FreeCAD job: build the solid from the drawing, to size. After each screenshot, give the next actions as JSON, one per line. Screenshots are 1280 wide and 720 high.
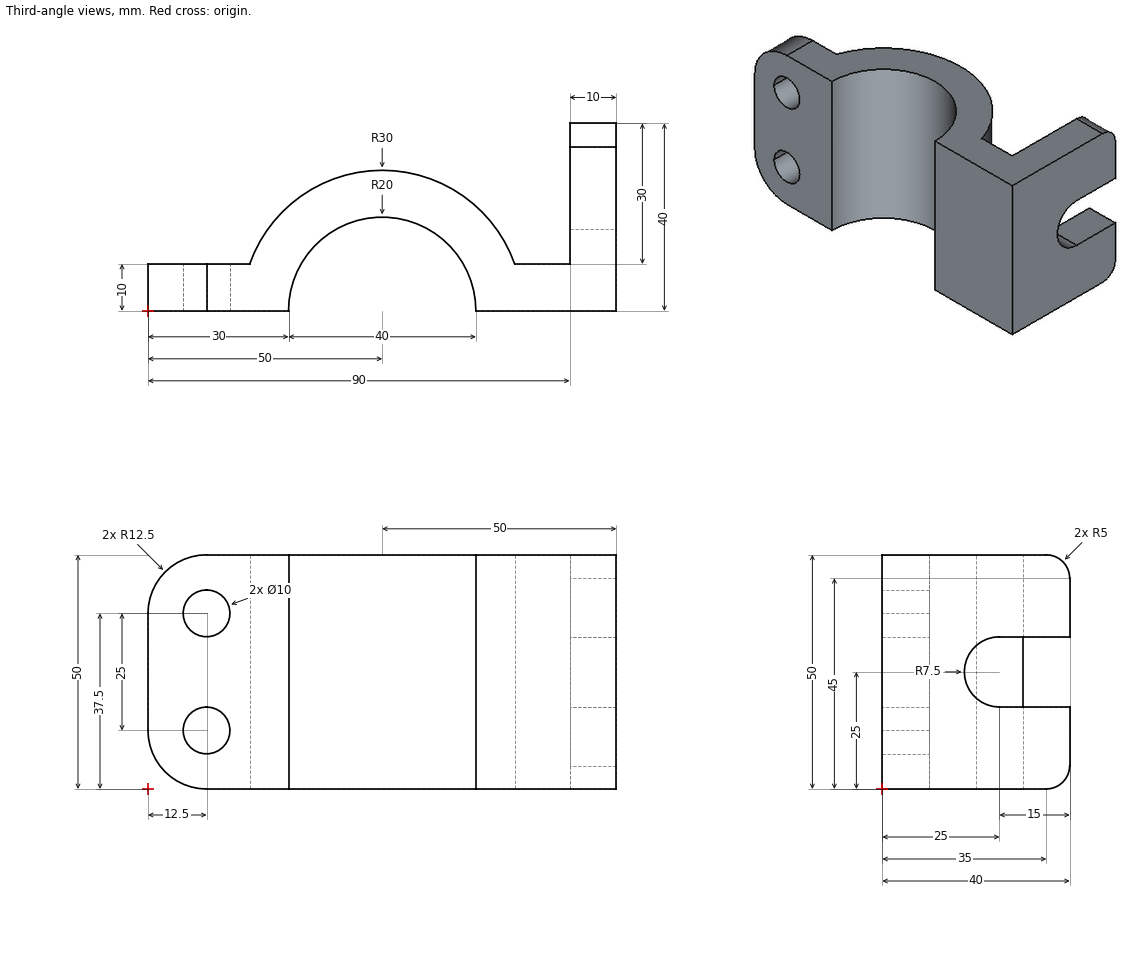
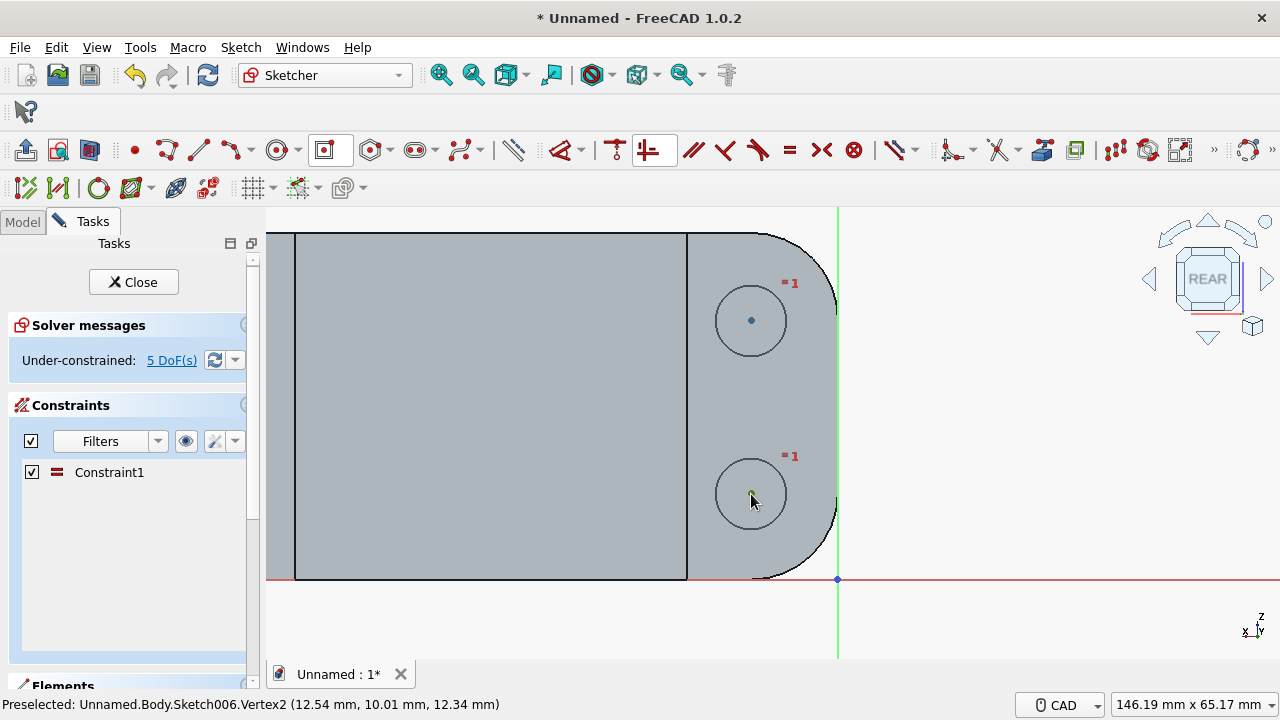
{"action": "key", "text": "v"}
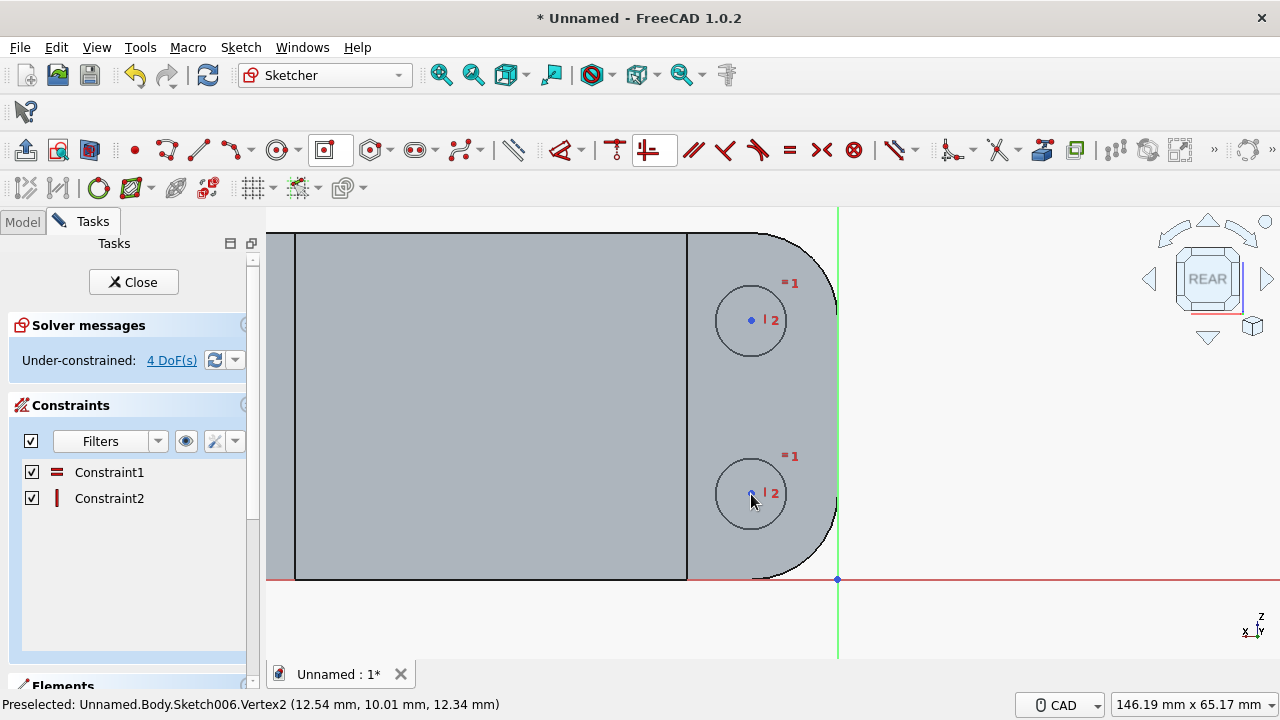
{"action": "left_click", "coordinate": [560, 150]}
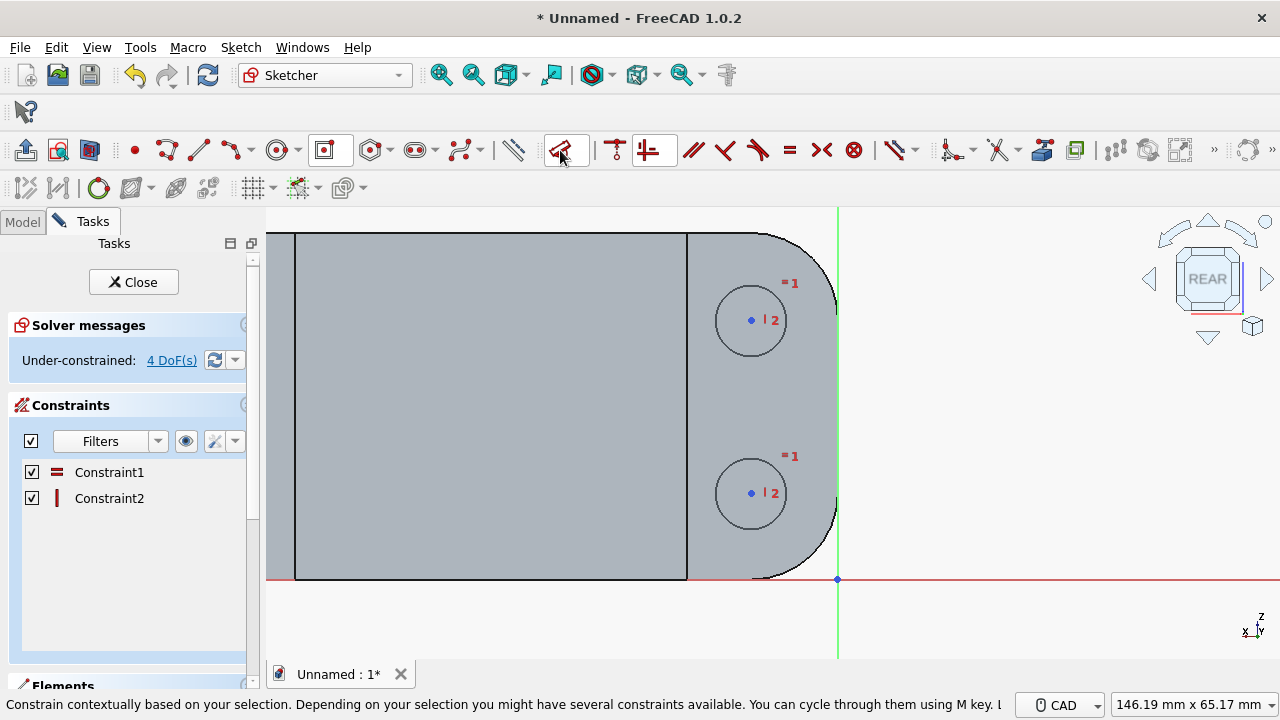
{"action": "left_click", "coordinate": [776, 296]}
{"action": "left_click", "coordinate": [799, 273]}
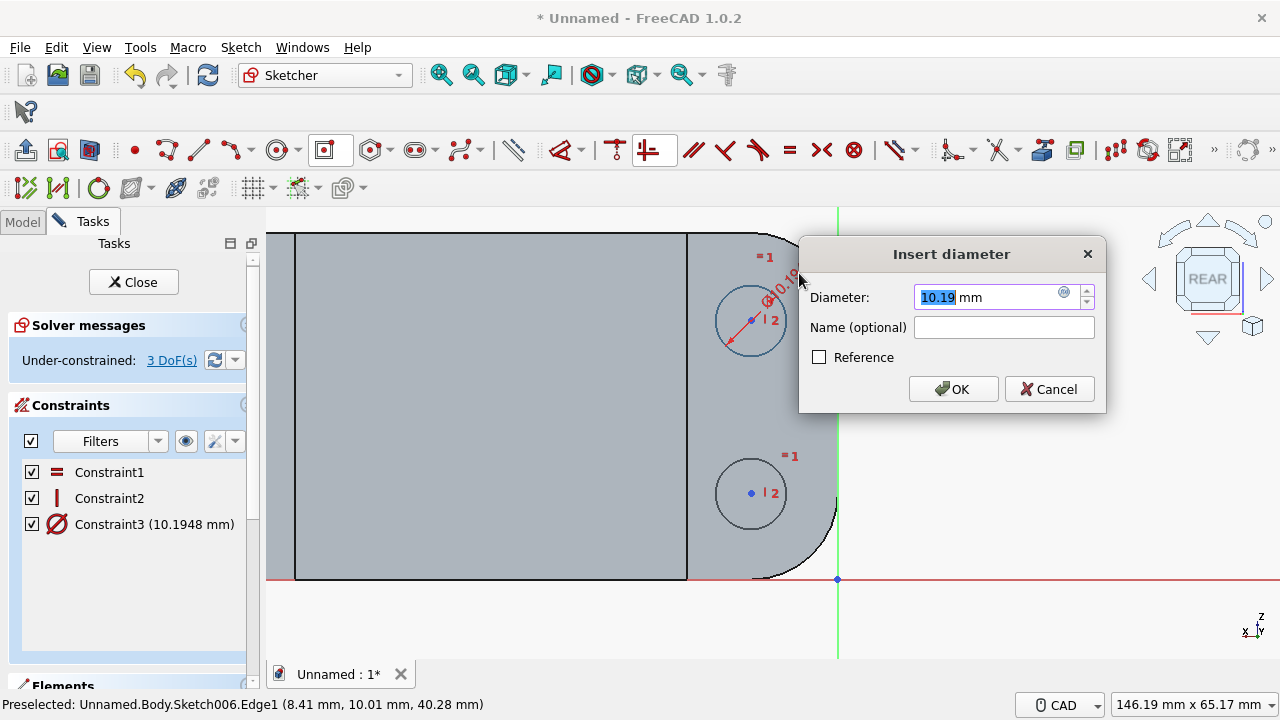
{"action": "type", "text": "10"}
{"action": "key", "text": "Return"}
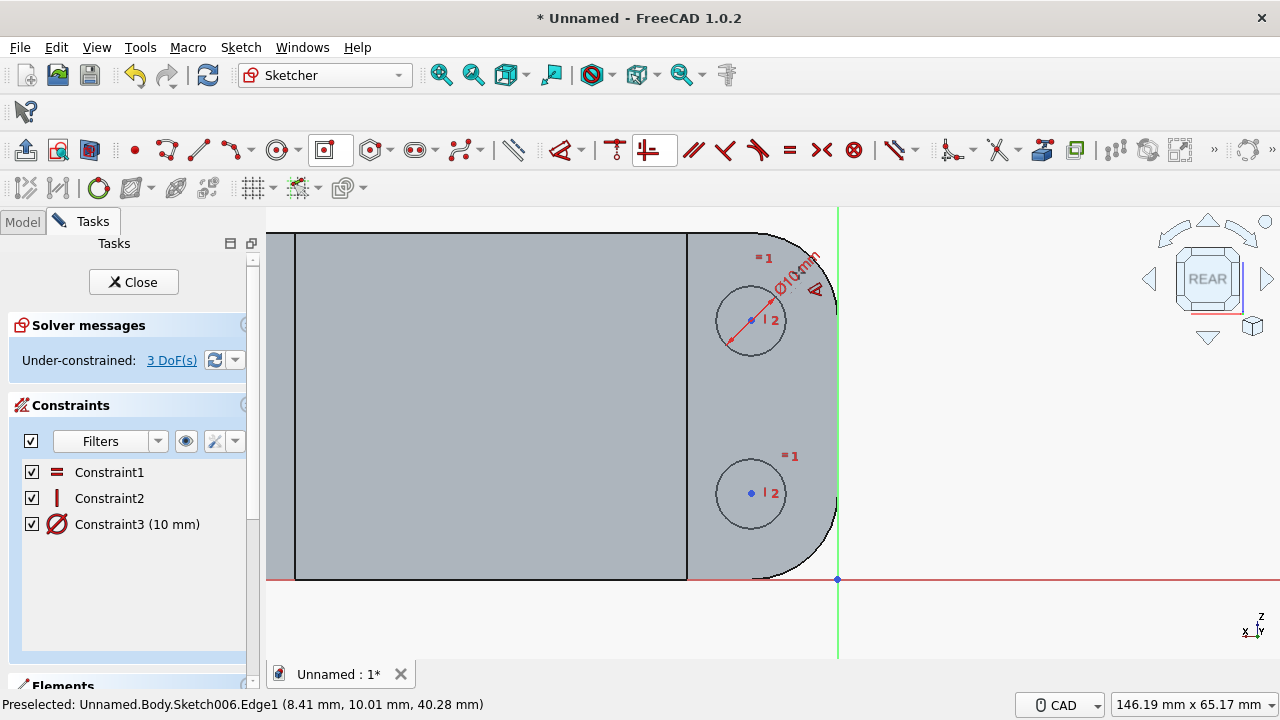
{"action": "left_click", "coordinate": [751, 321]}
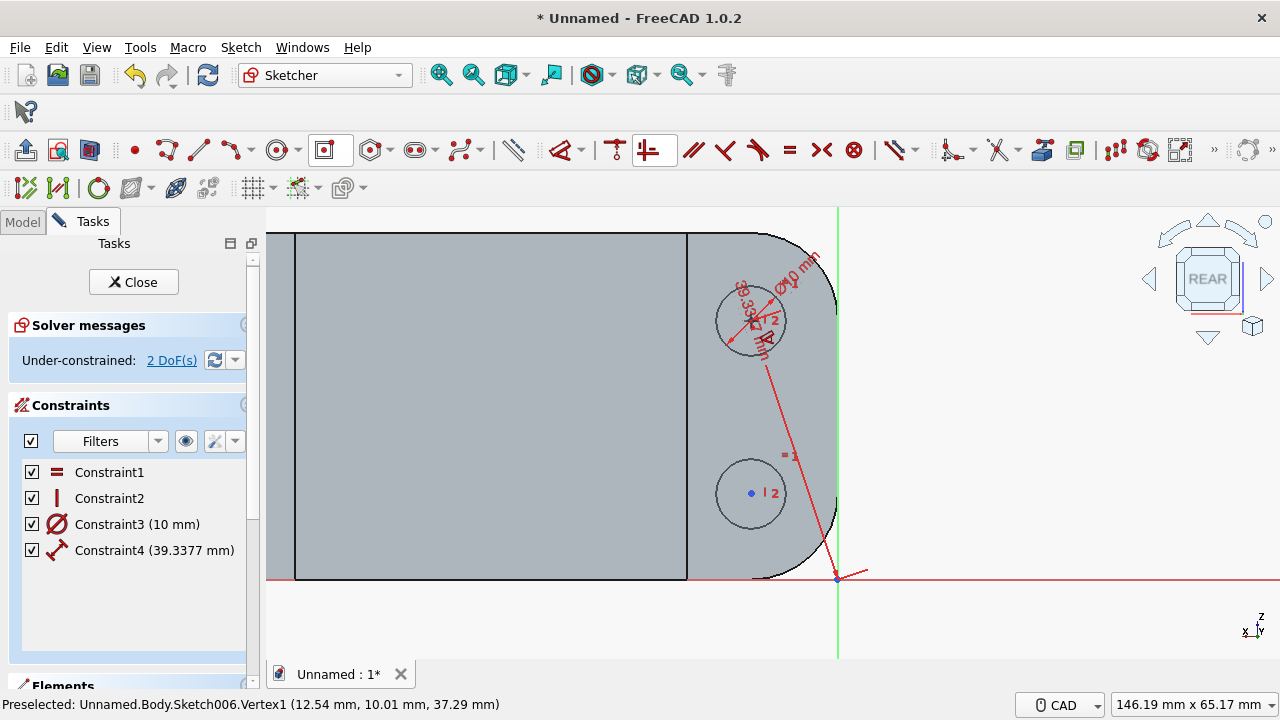
{"action": "left_click", "coordinate": [751, 494]}
{"action": "left_click", "coordinate": [717, 408]}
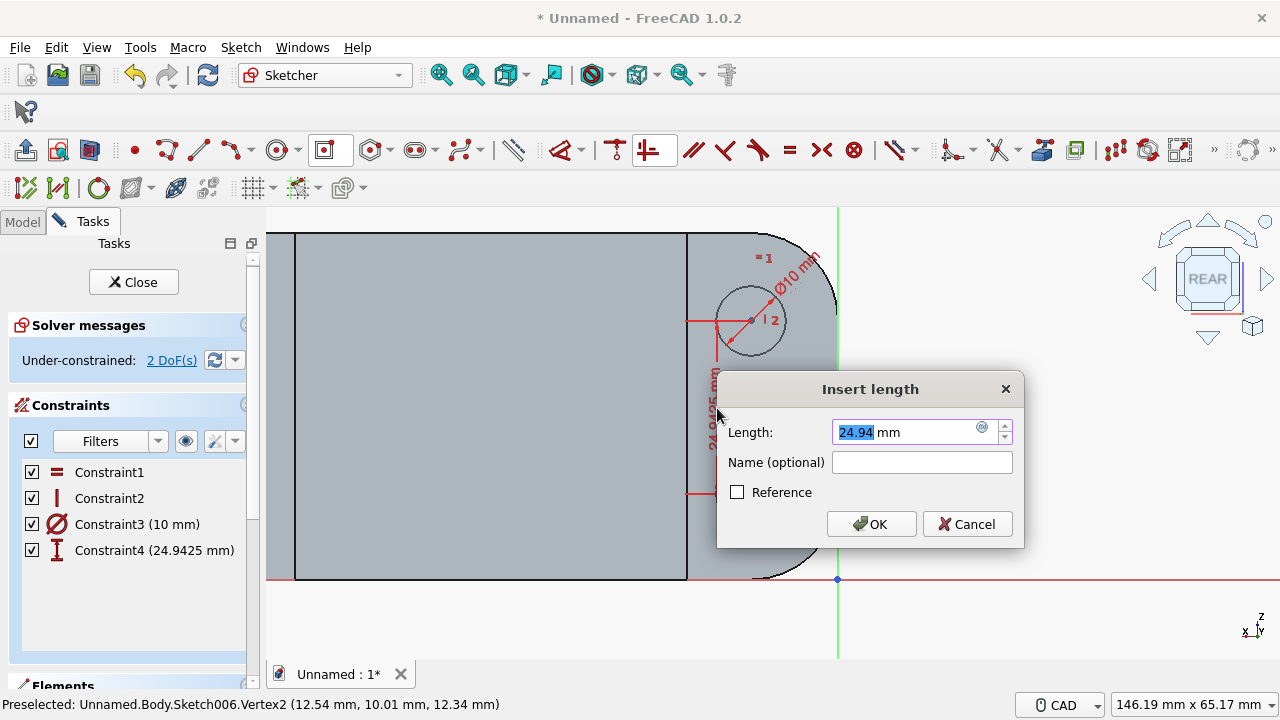
{"action": "type", "text": "25"}
{"action": "key", "text": "Return"}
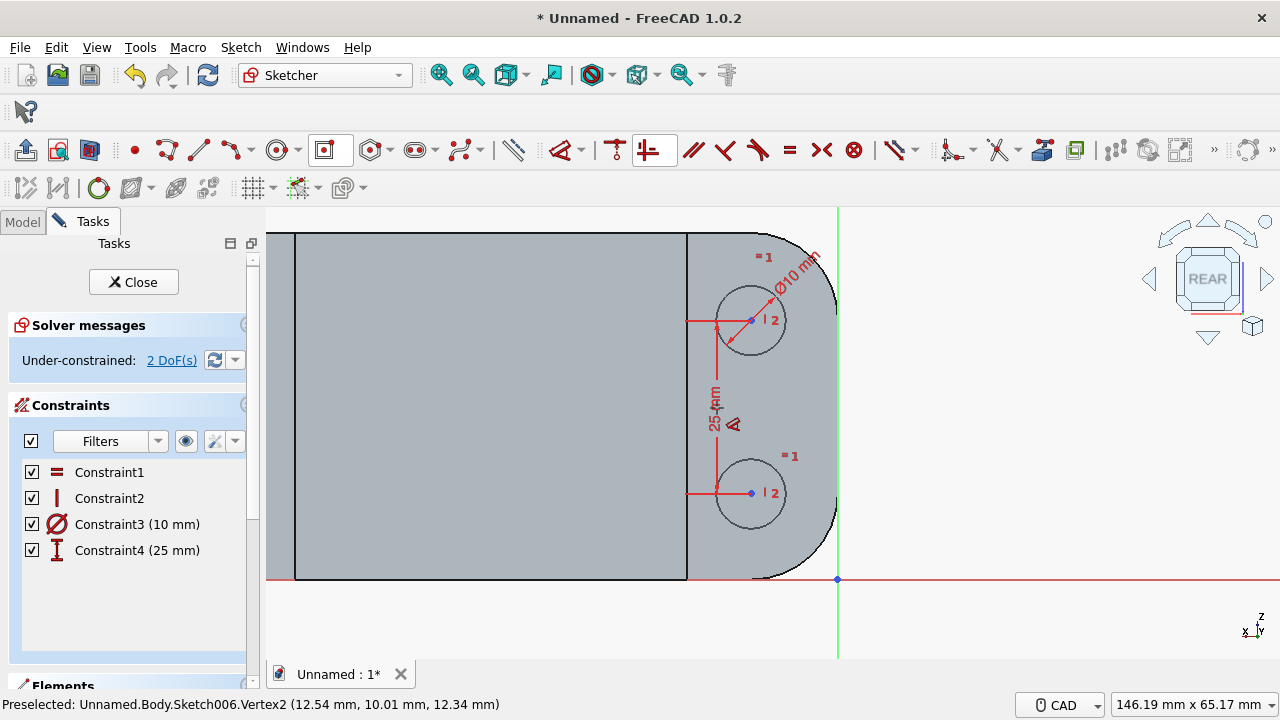
{"action": "left_click", "coordinate": [751, 321]}
{"action": "left_click", "coordinate": [794, 614]}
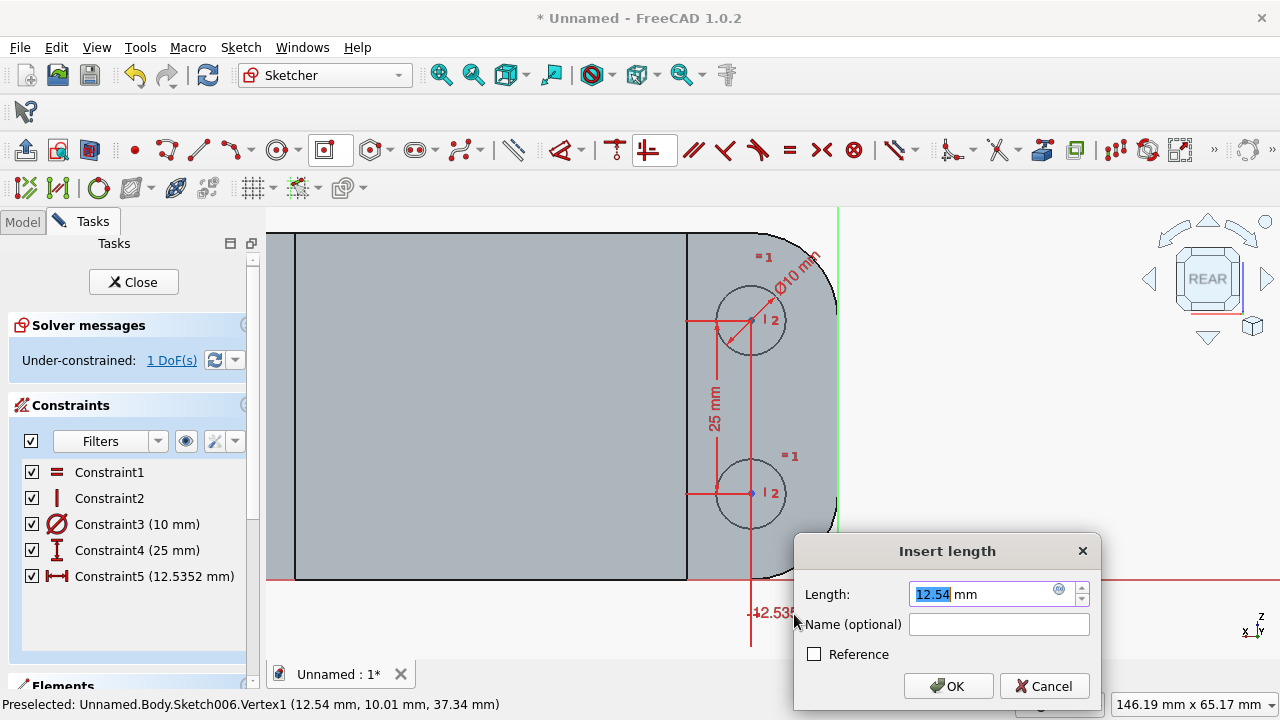
{"action": "type", "text": "12.5"}
{"action": "key", "text": "Return"}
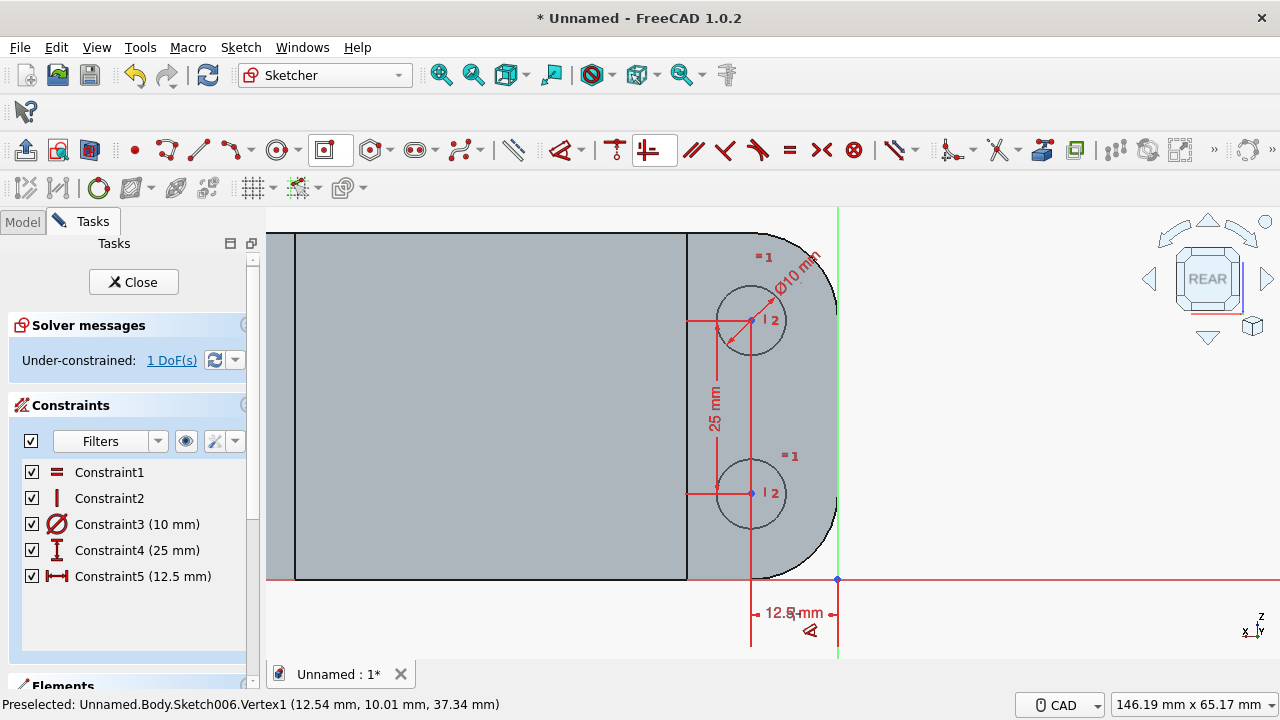
{"action": "left_click", "coordinate": [751, 321]}
{"action": "left_click", "coordinate": [872, 450]}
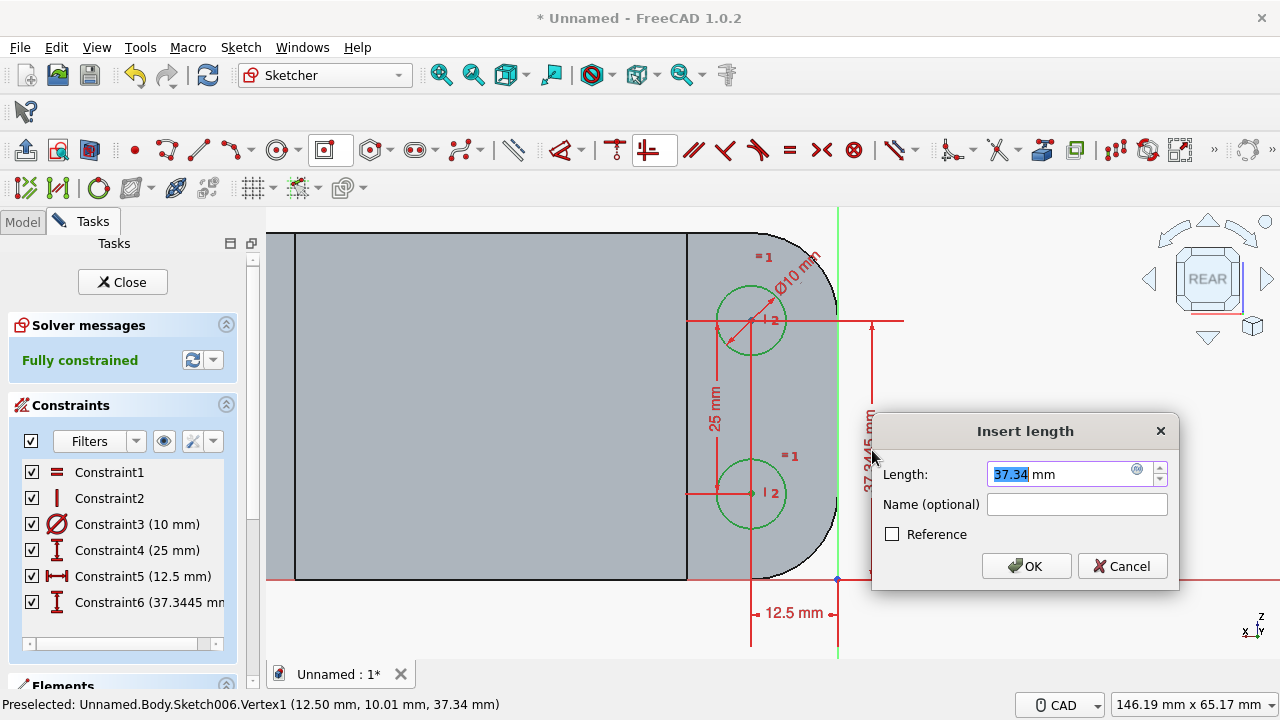
{"action": "type", "text": "37.5"}
{"action": "key", "text": "Return"}
{"action": "key", "text": "Escape"}